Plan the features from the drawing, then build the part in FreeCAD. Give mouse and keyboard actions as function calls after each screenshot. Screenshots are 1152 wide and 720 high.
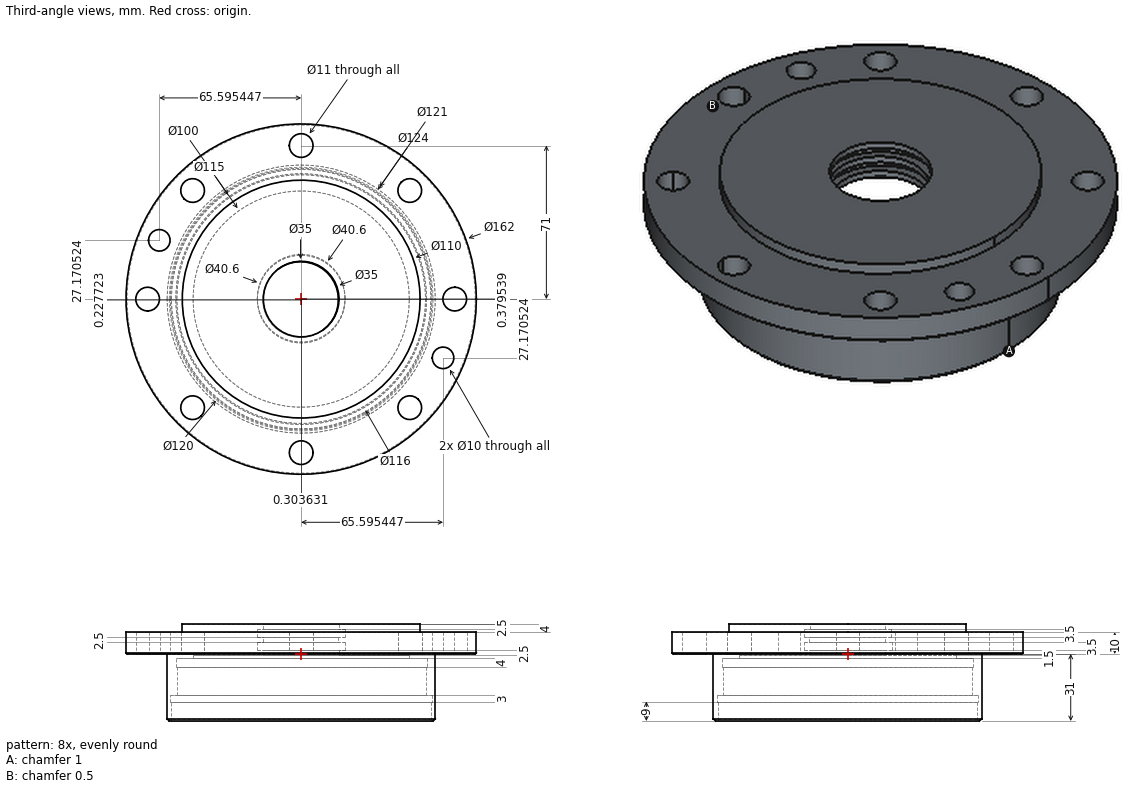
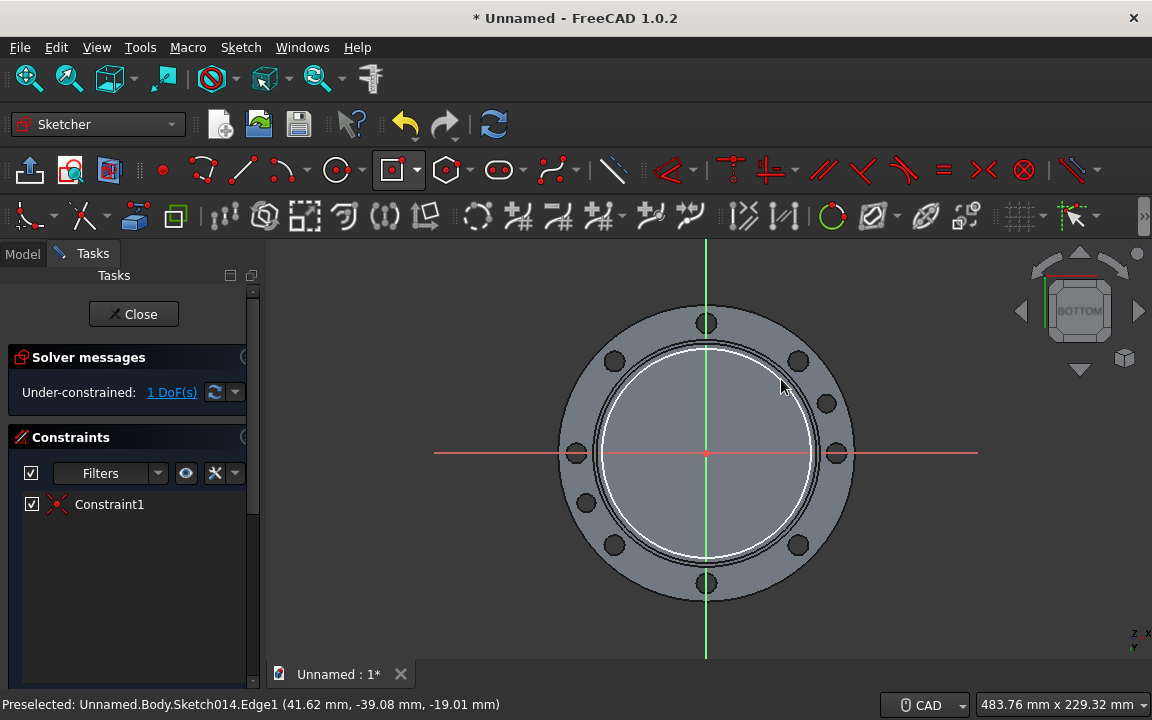
click(668, 170)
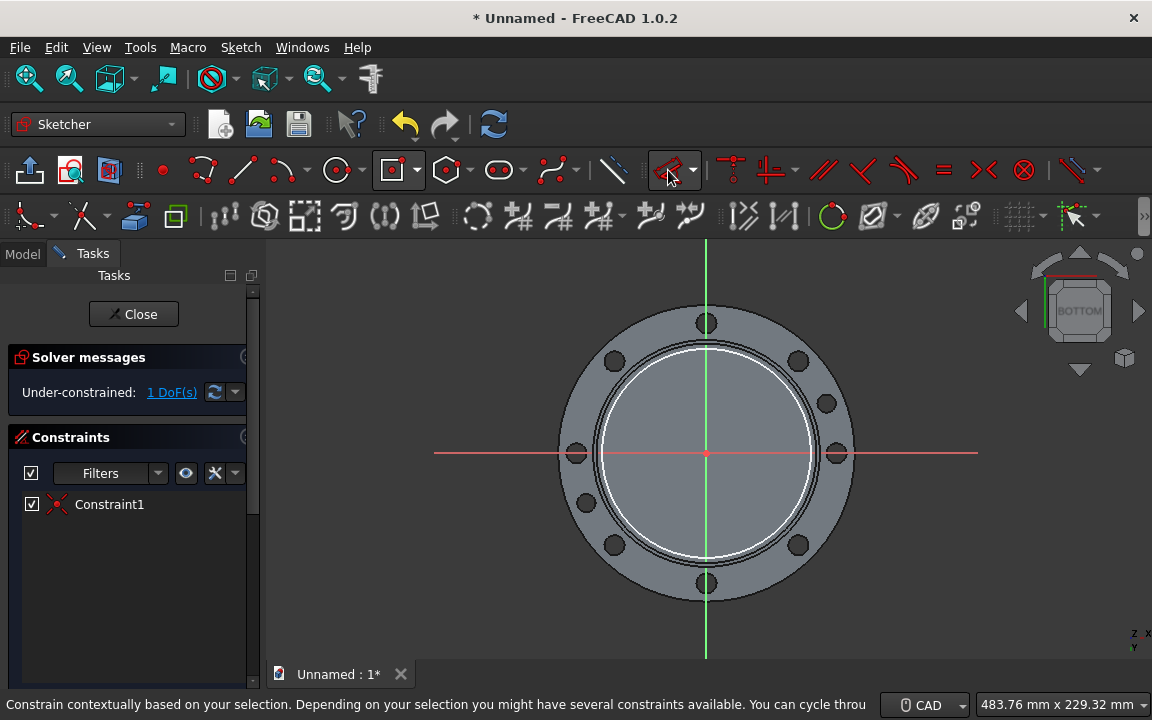
click(780, 379)
click(802, 356)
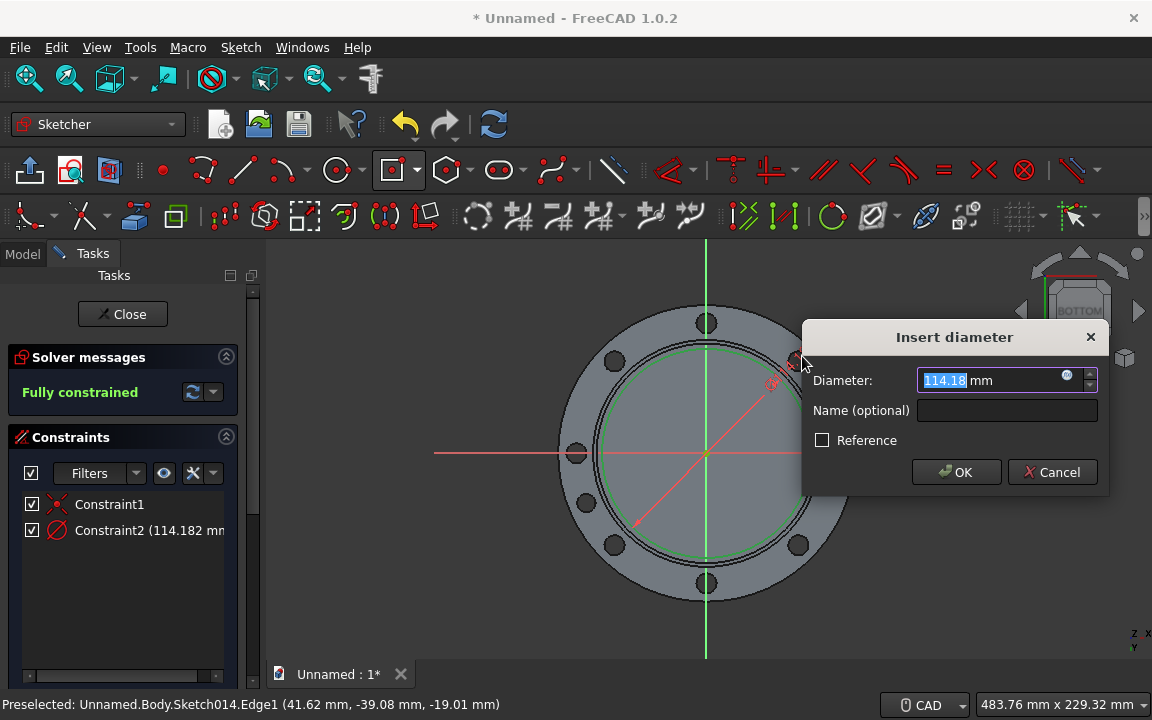
text(115)
key(Return)
key(Escape)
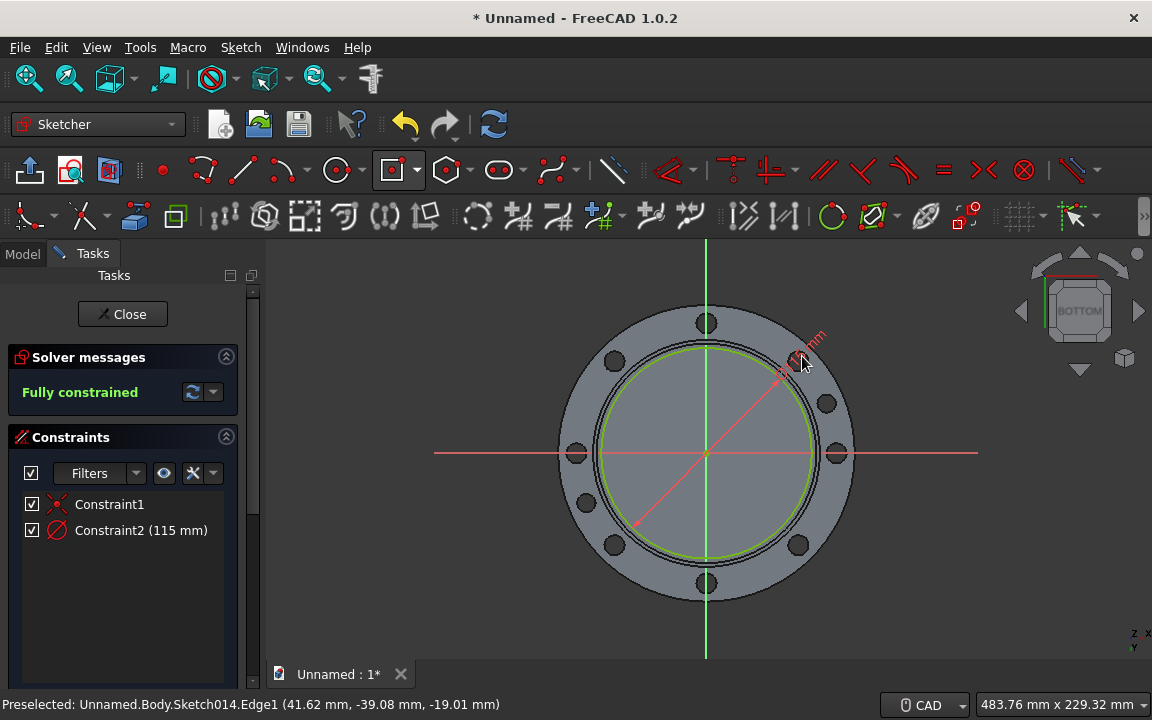
click(123, 314)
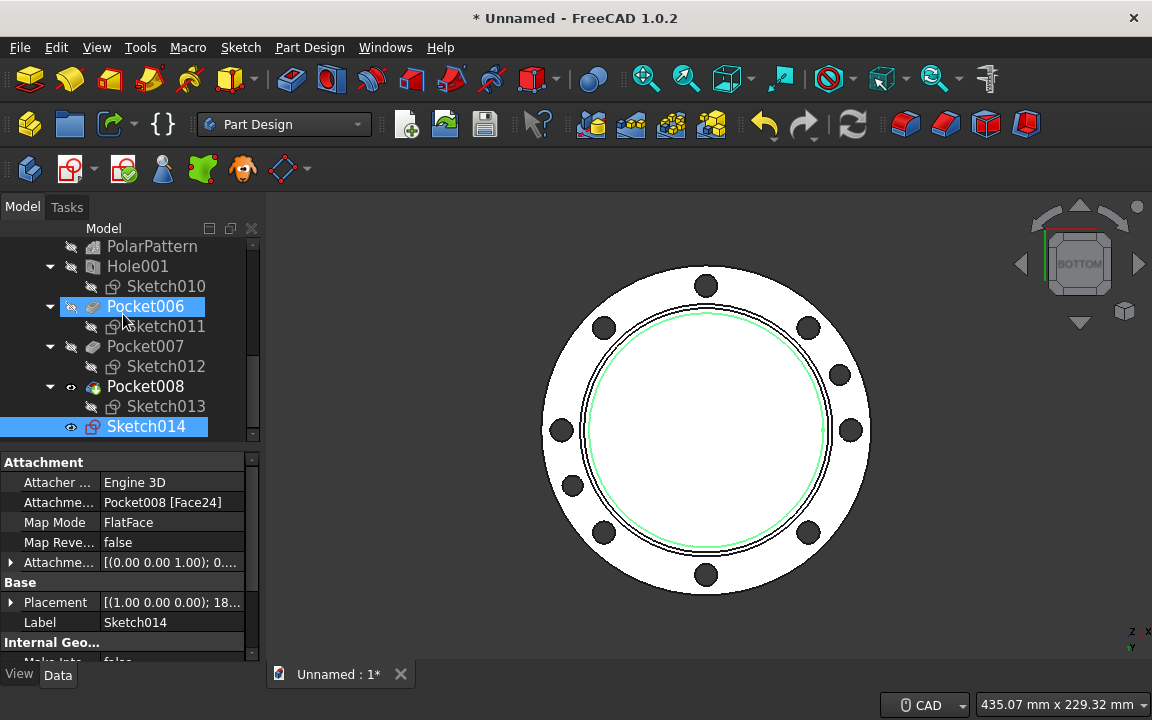
click(292, 80)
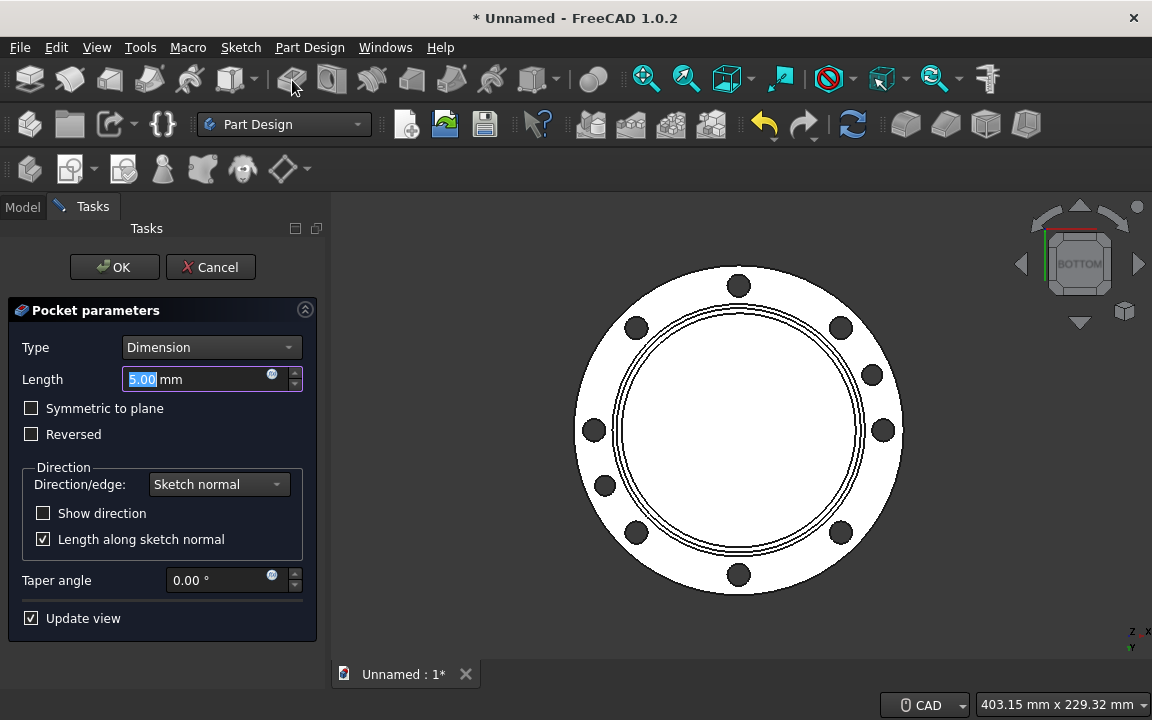
click(212, 348)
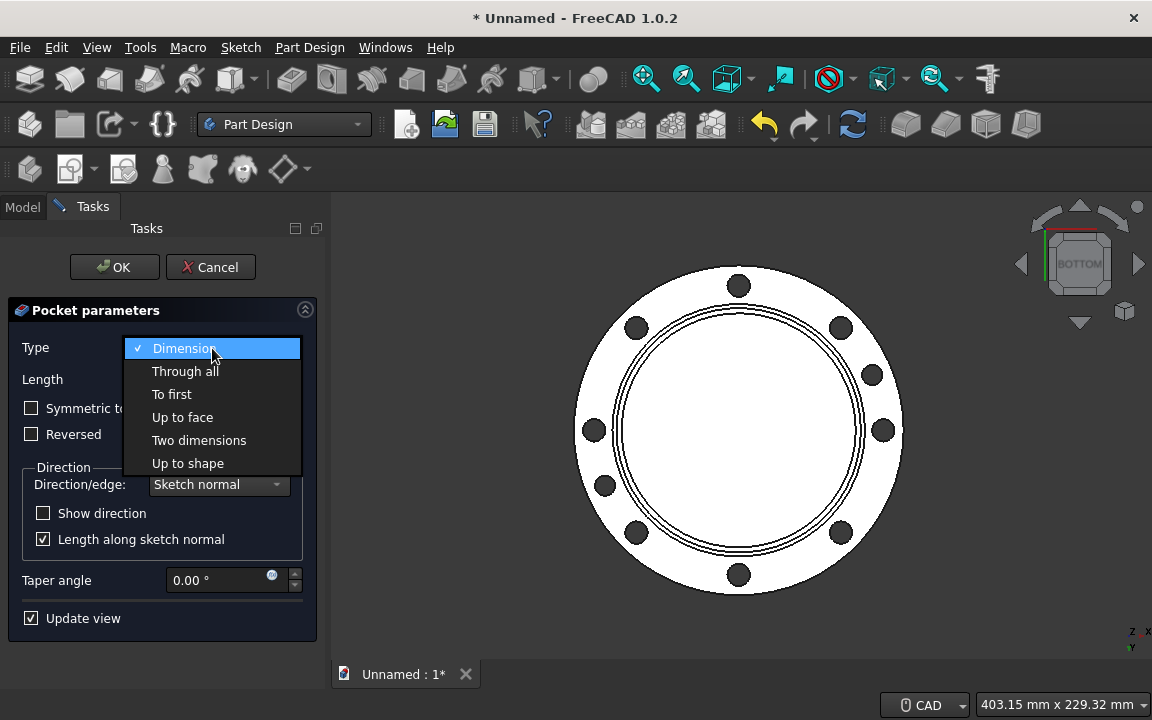
click(212, 394)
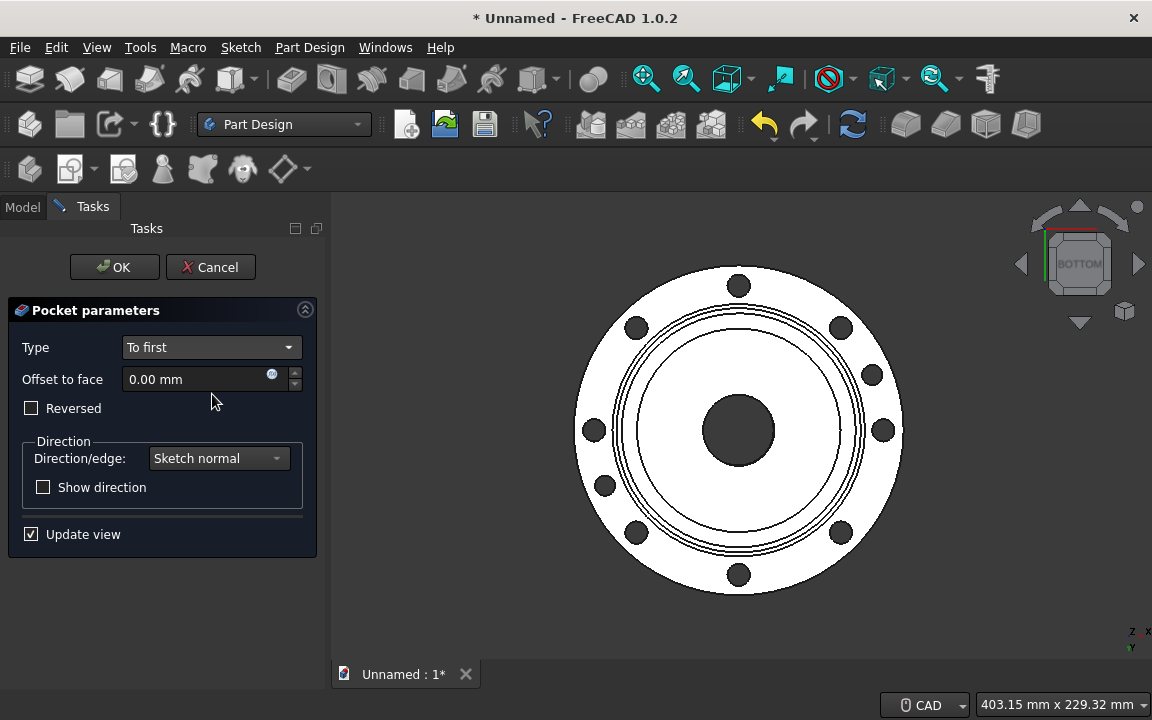
click(115, 267)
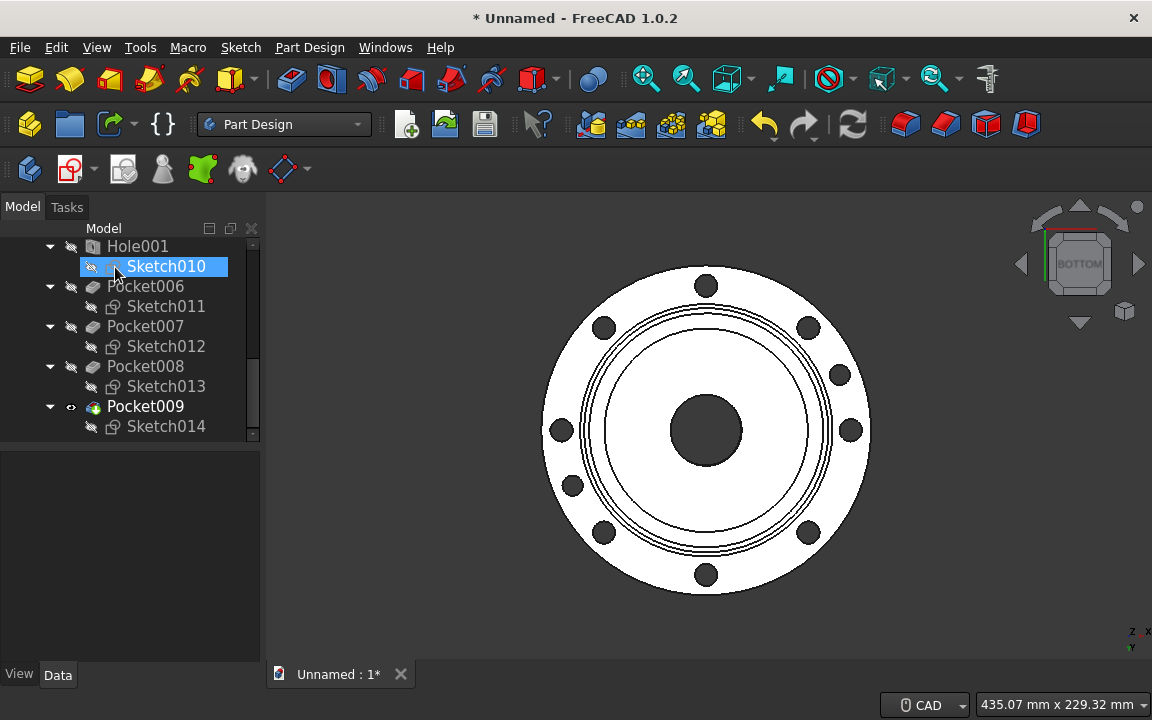
key(0)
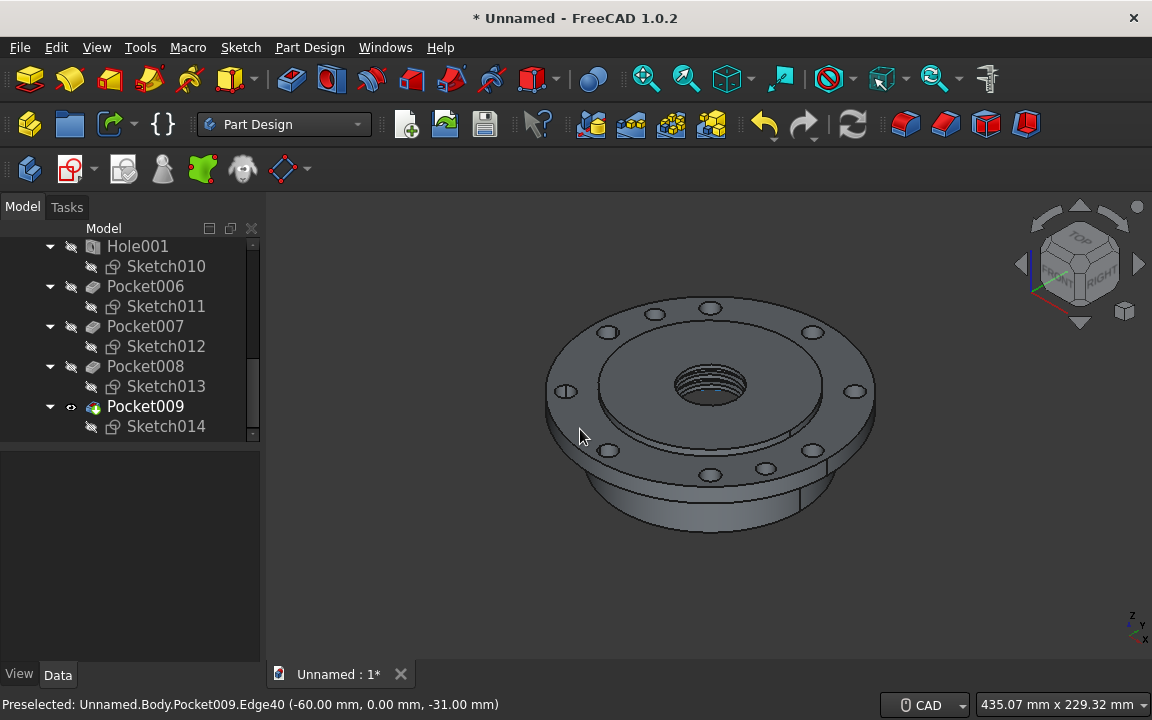
key(2)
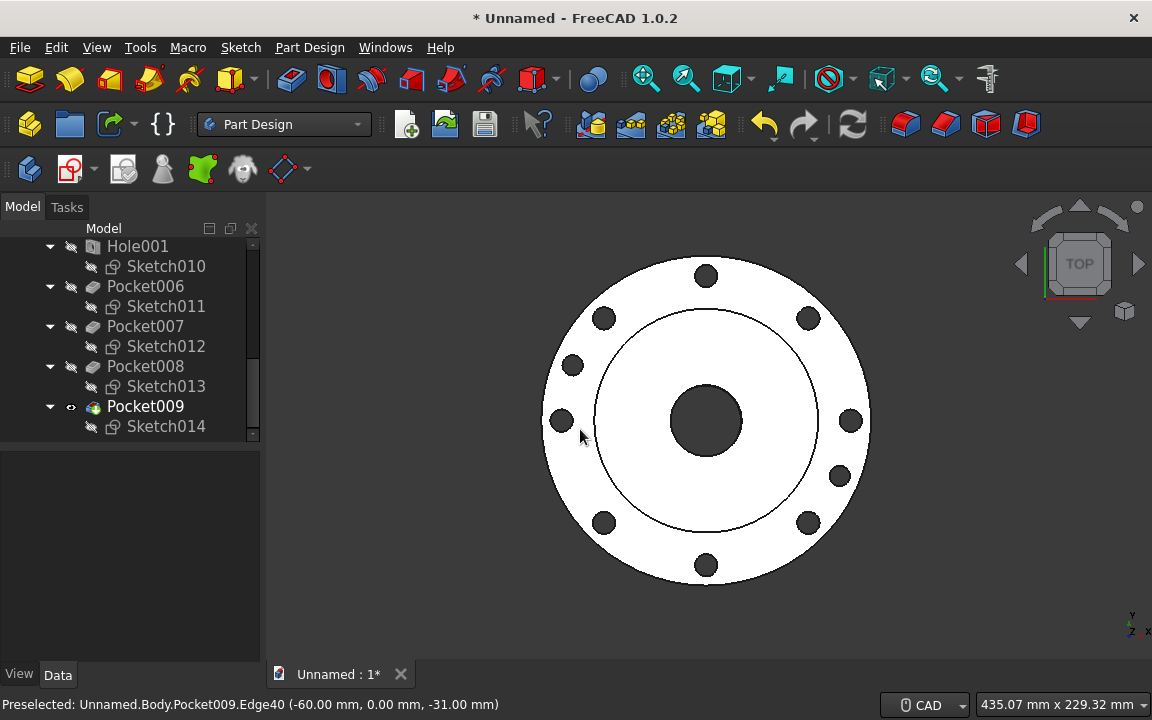
key(1)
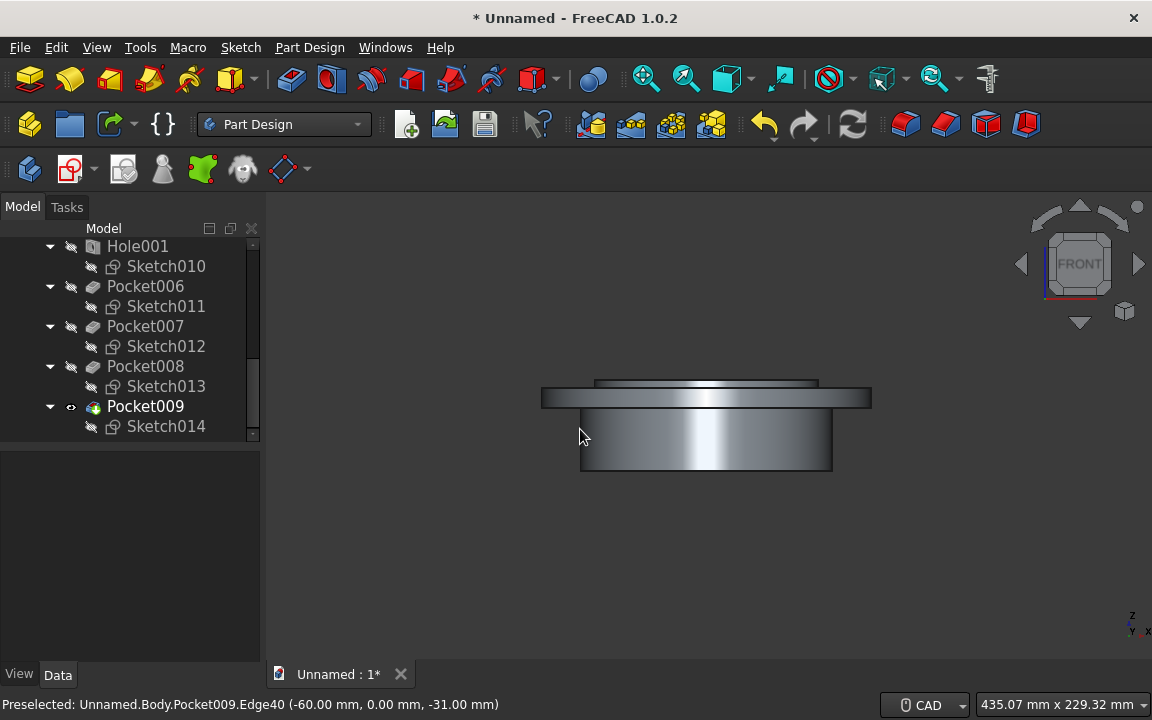
click(648, 80)